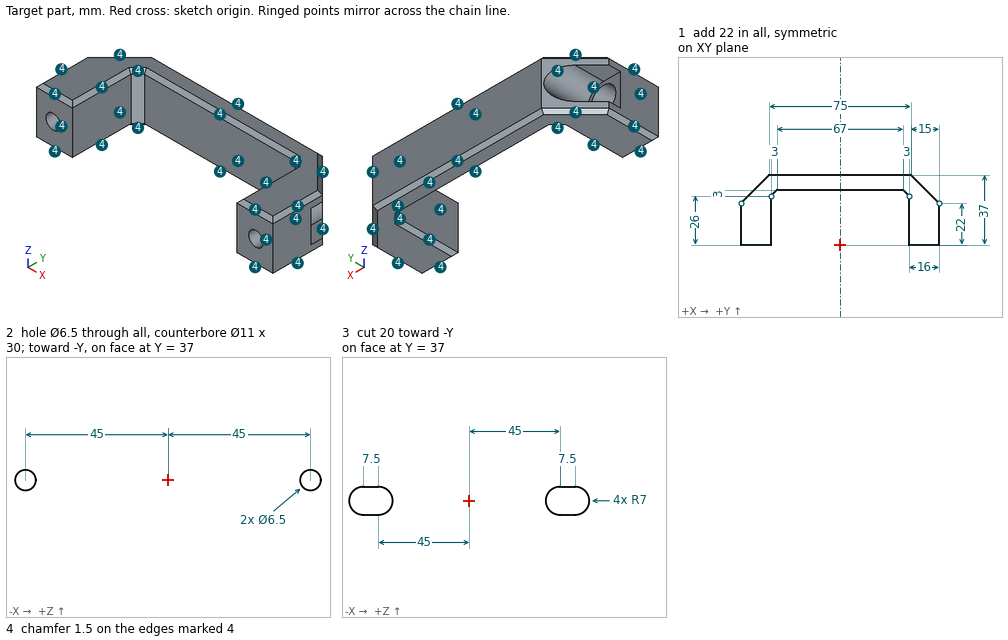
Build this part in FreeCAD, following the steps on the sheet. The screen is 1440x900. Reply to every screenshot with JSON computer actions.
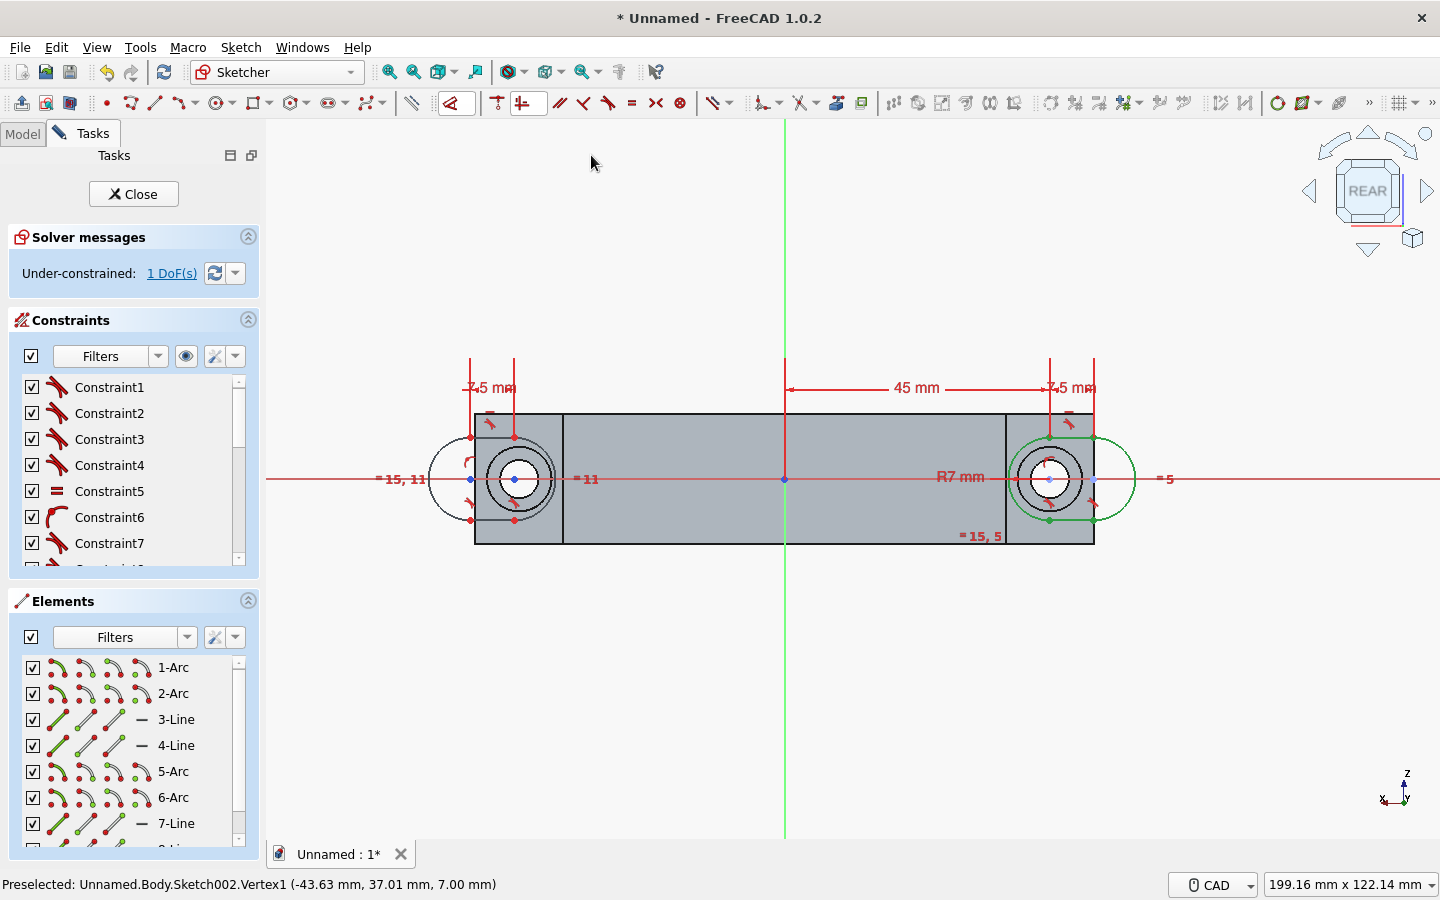
{"action": "left_click", "coordinate": [514, 520]}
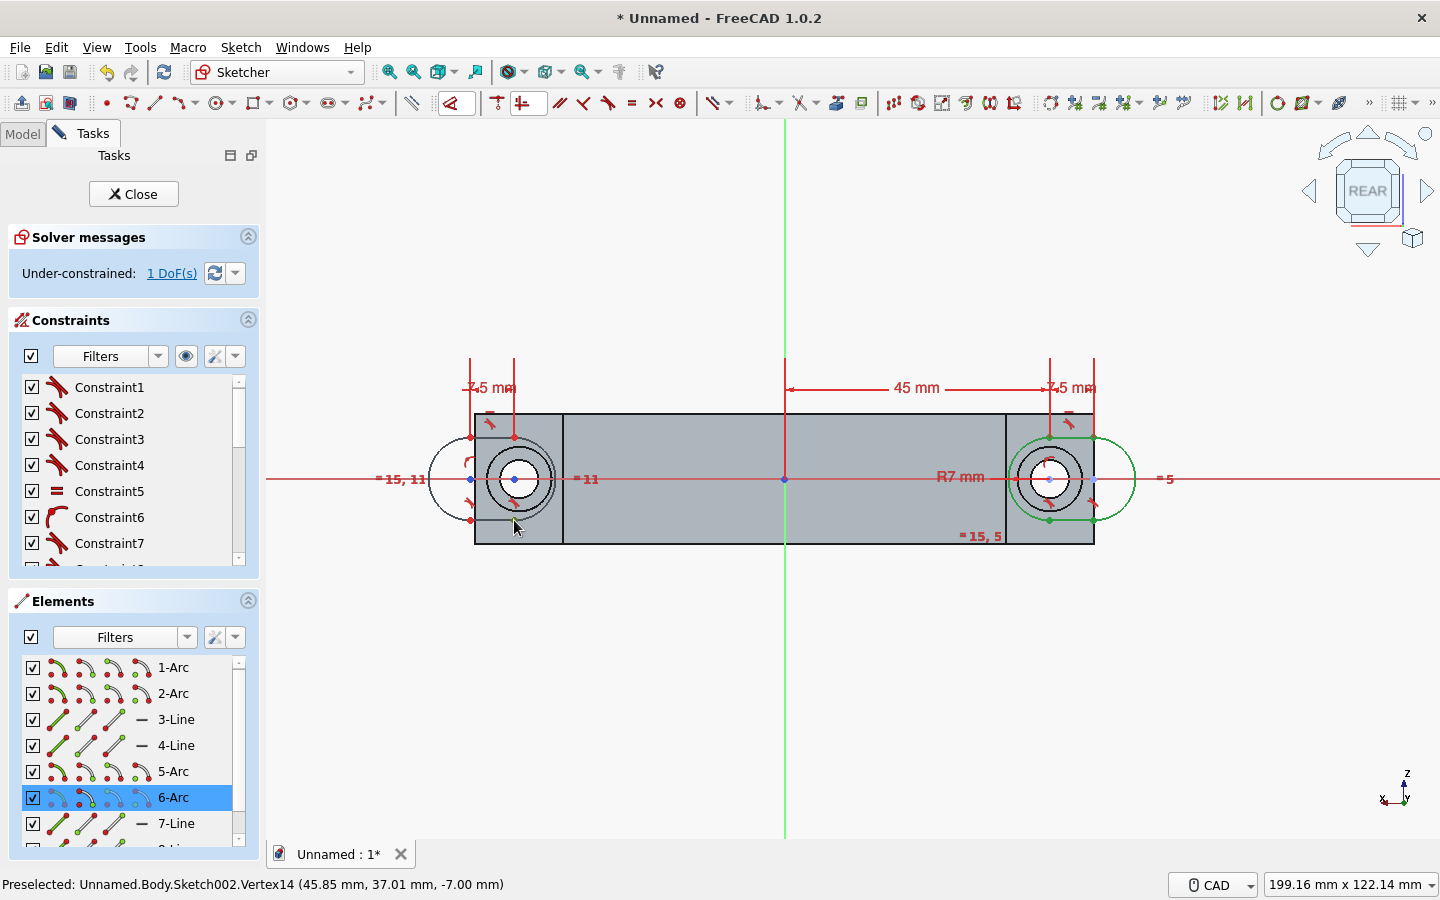
{"action": "left_click", "coordinate": [470, 104]}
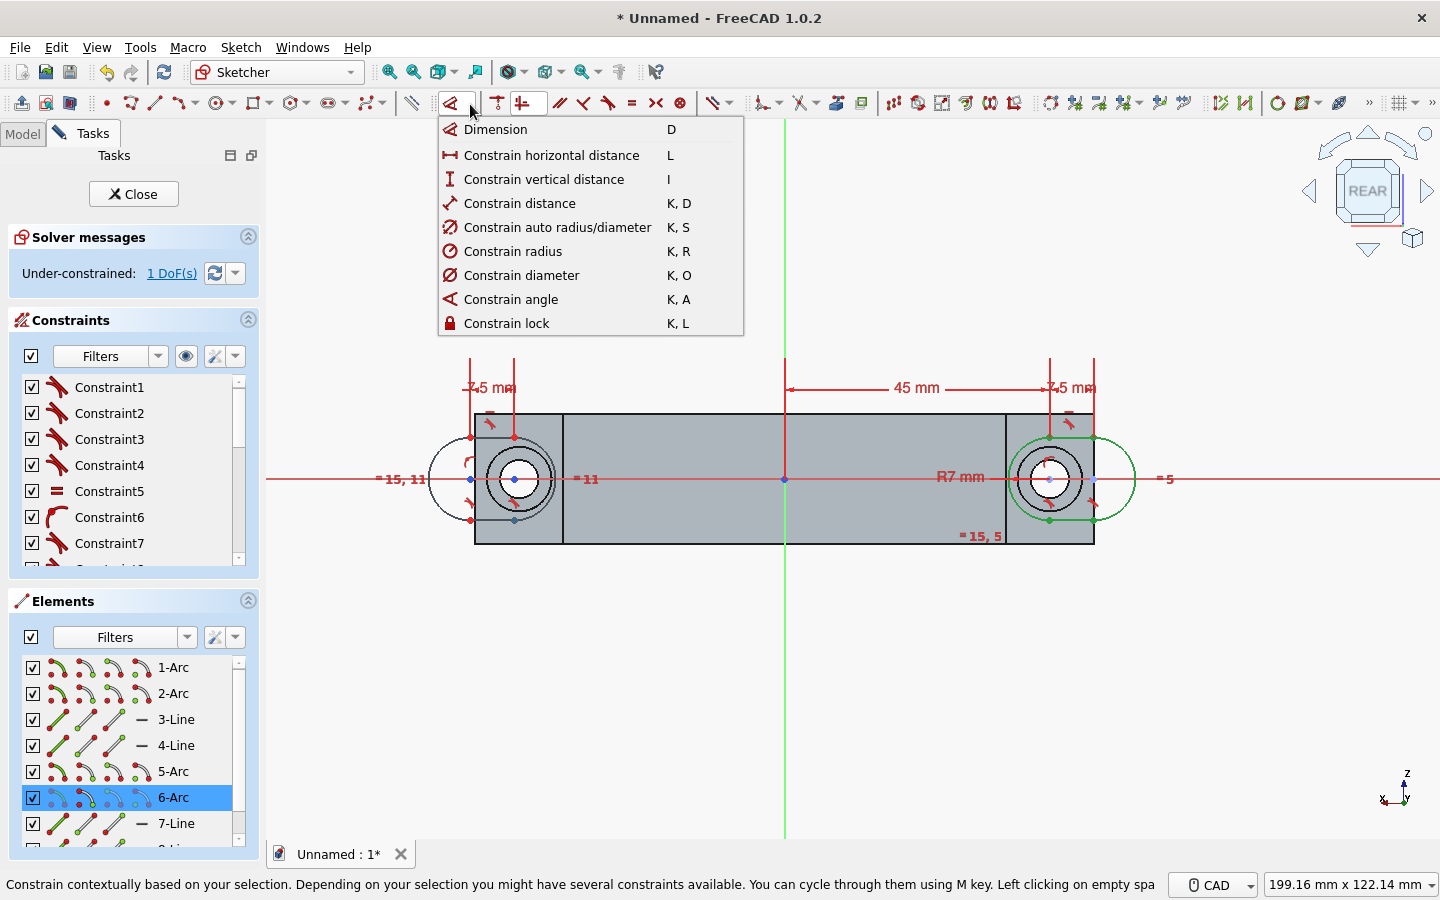
{"action": "left_click", "coordinate": [591, 155]}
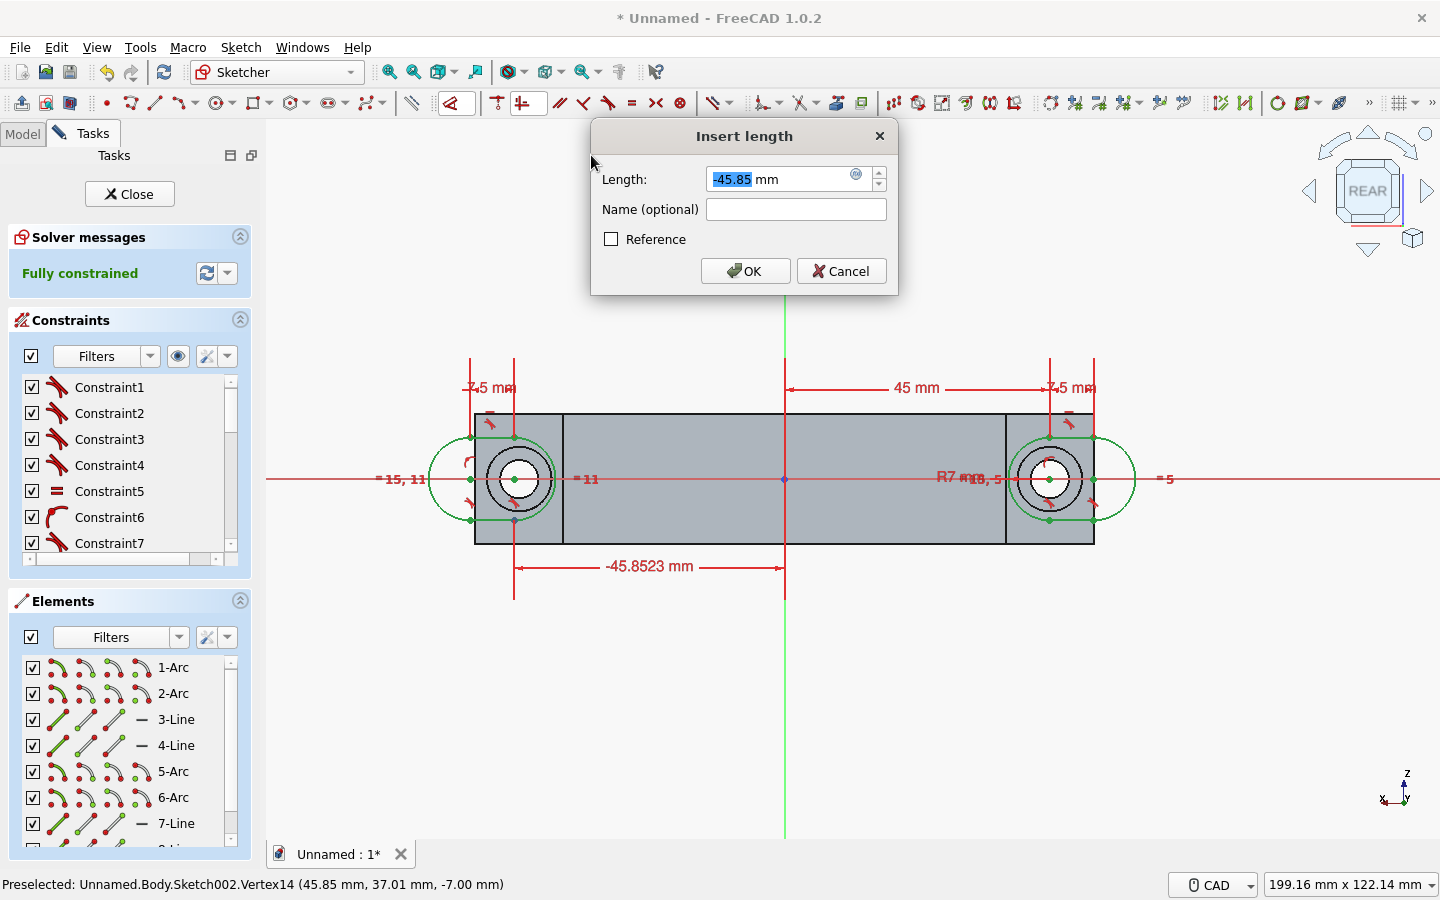
{"action": "type", "text": "-45"}
{"action": "key", "text": "Return"}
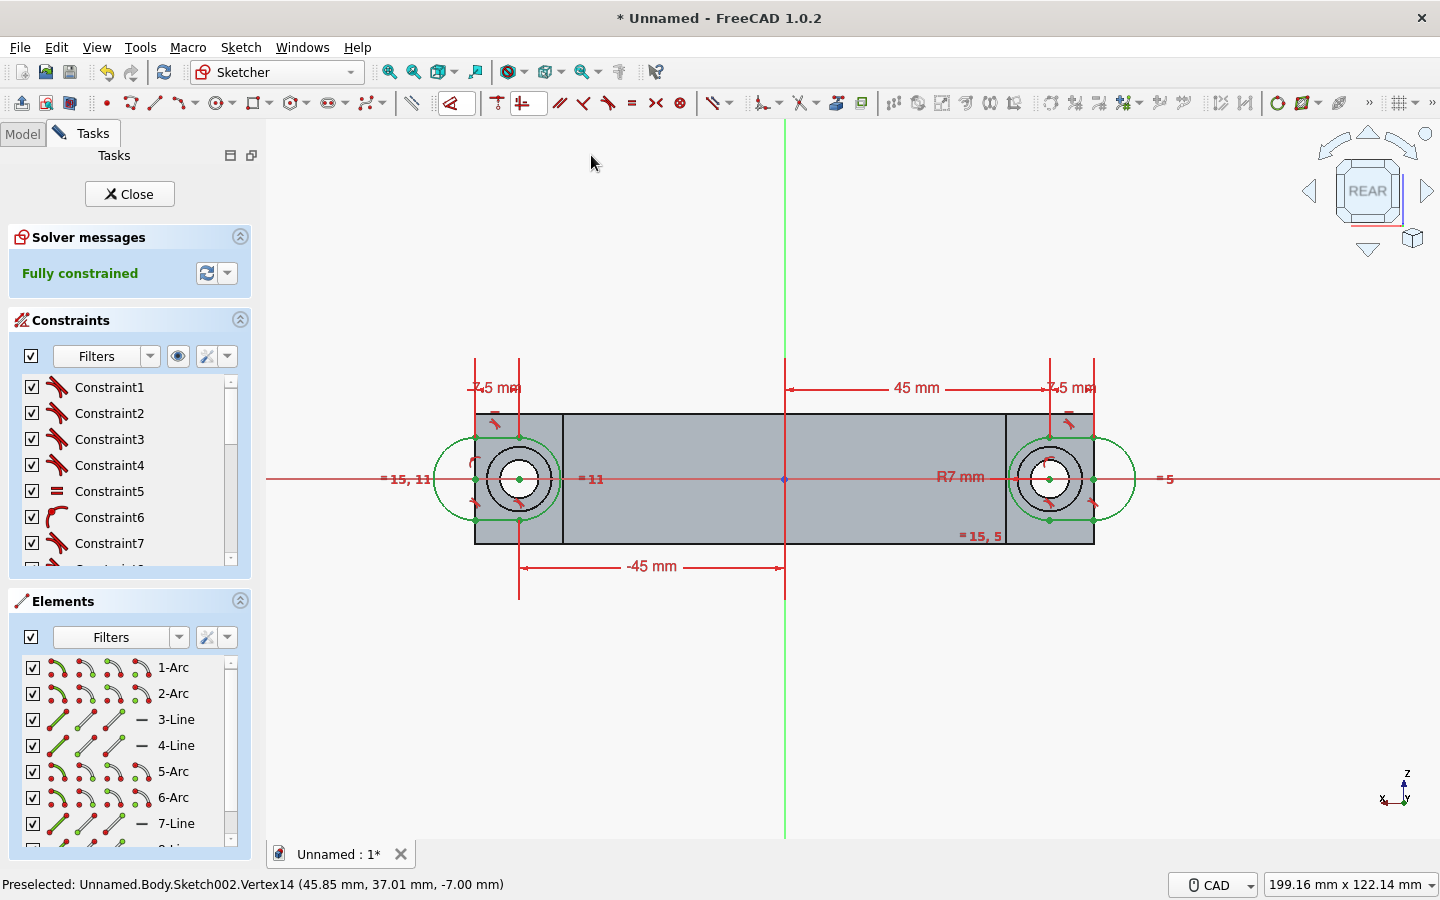
{"action": "left_click", "coordinate": [130, 194]}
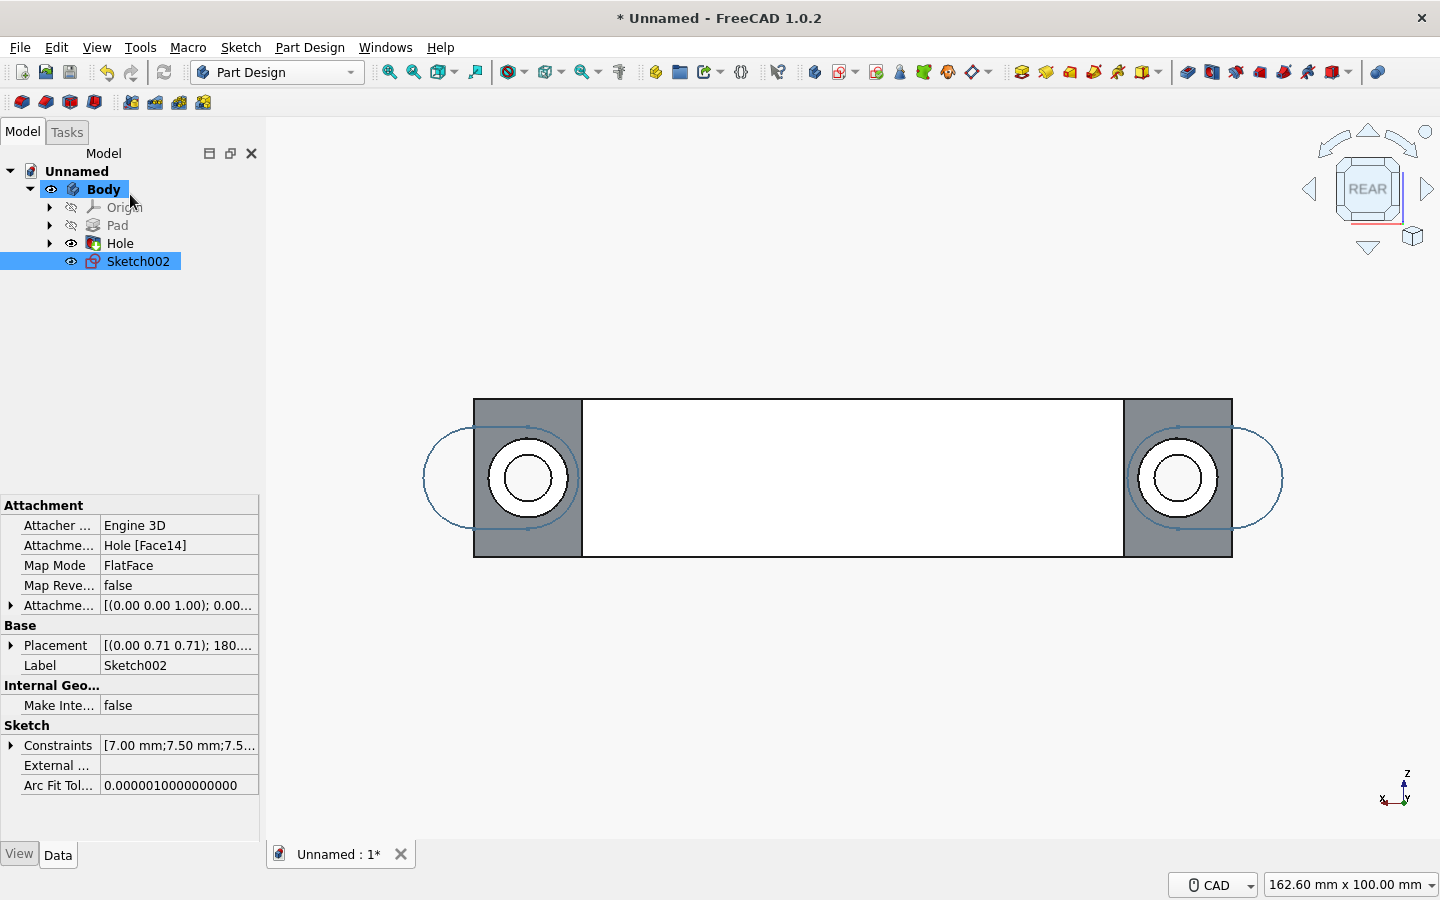
{"action": "left_click", "coordinate": [1188, 72]}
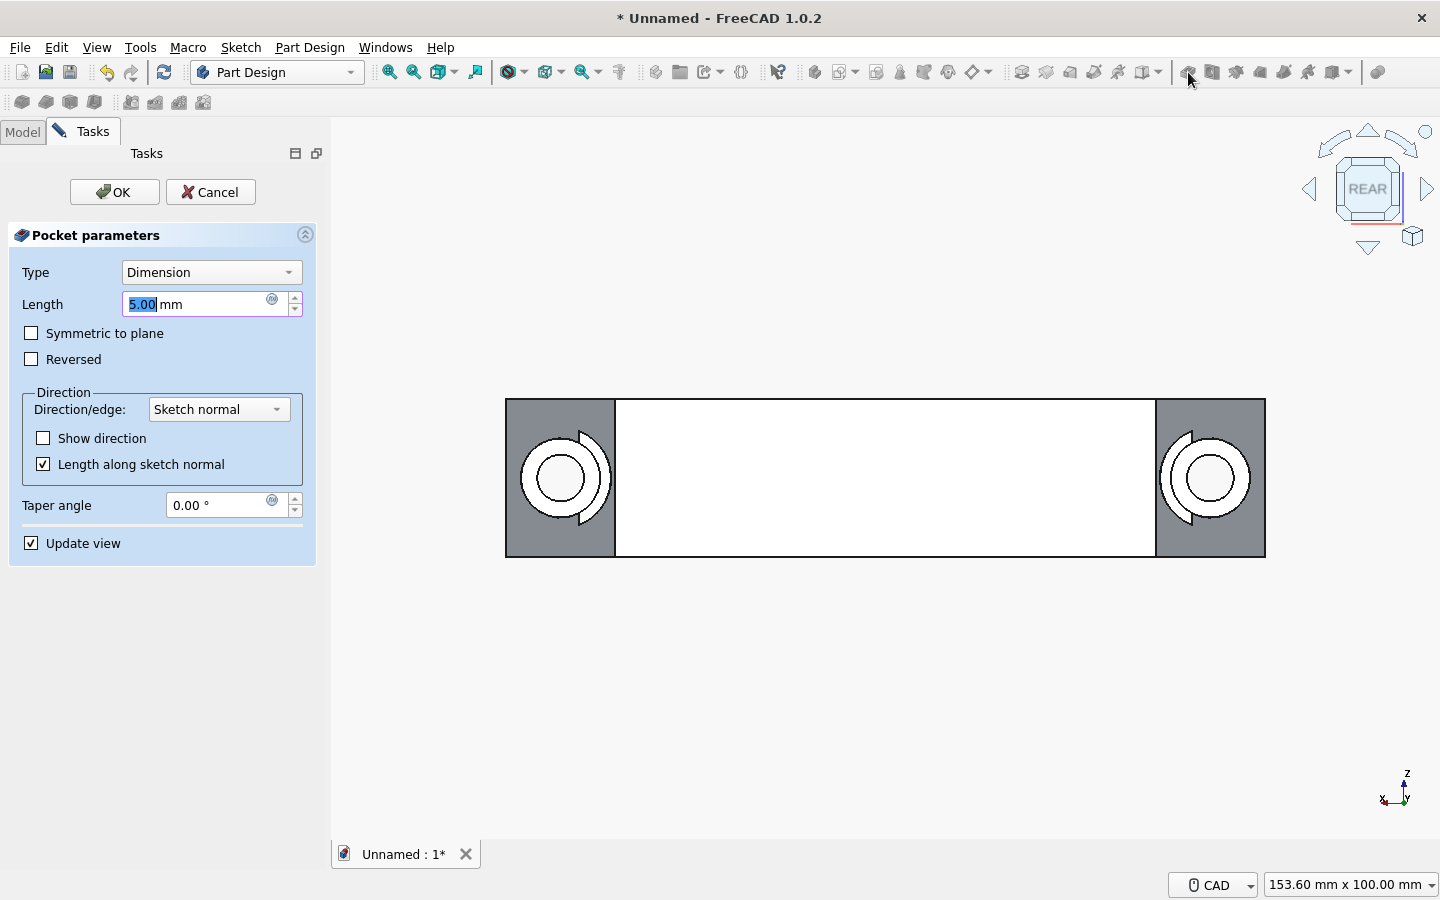
{"action": "type", "text": "20"}
{"action": "key", "text": "Tab"}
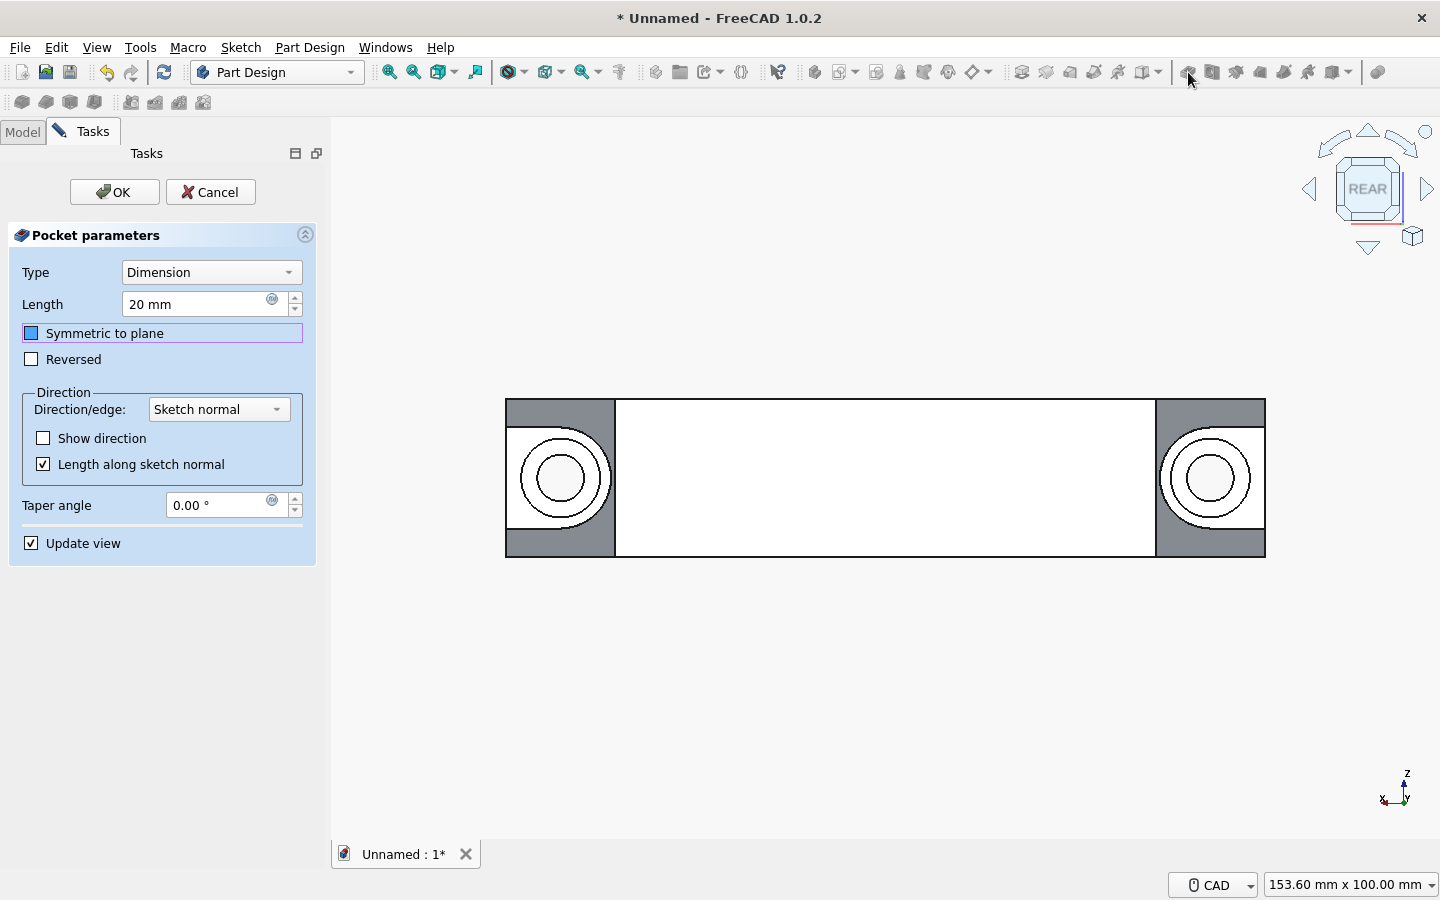
{"action": "left_click", "coordinate": [115, 192]}